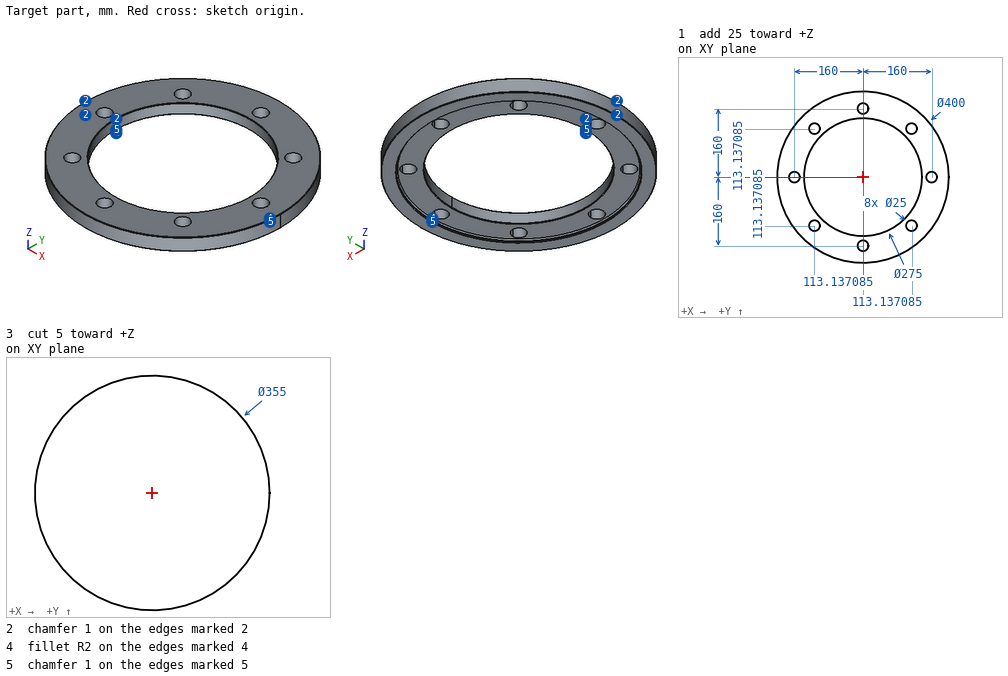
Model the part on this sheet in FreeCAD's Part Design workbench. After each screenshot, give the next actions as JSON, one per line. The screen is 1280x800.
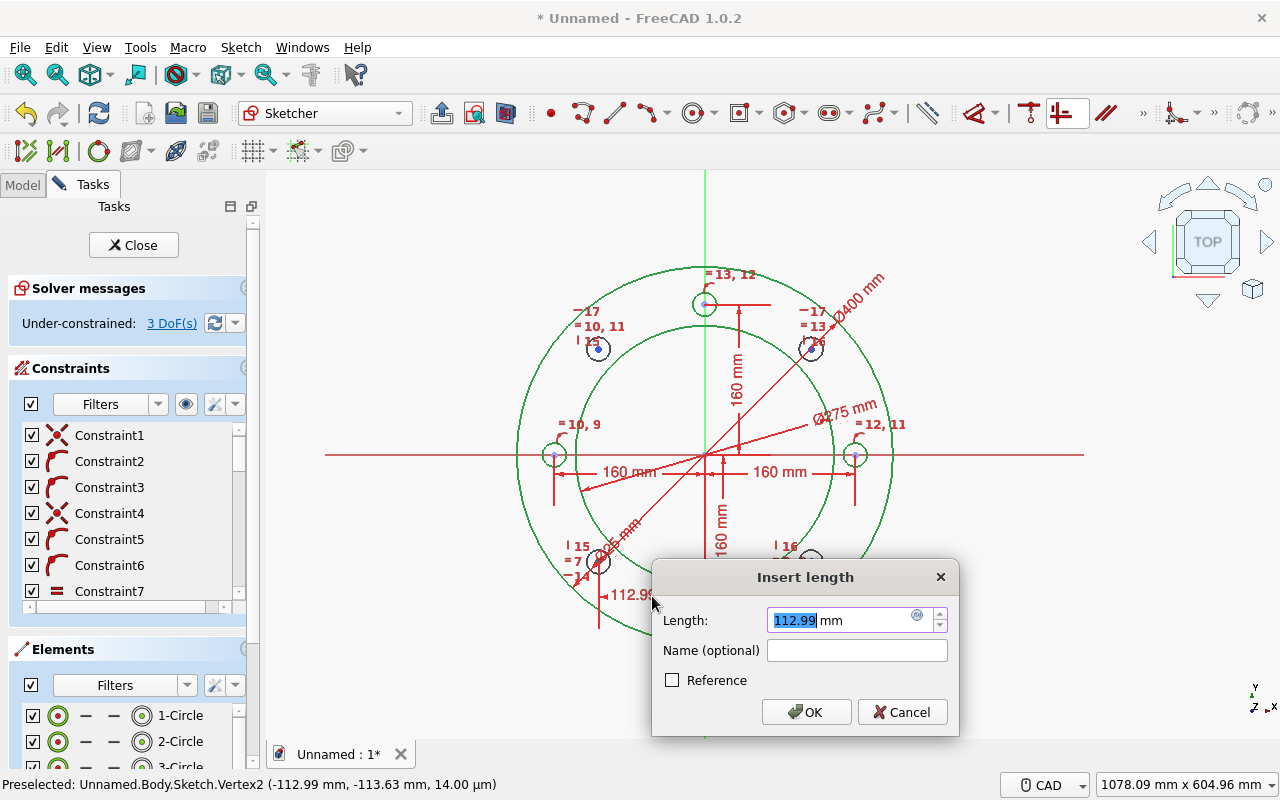
{"action": "type", "text": "113.137085"}
{"action": "key", "text": "Return"}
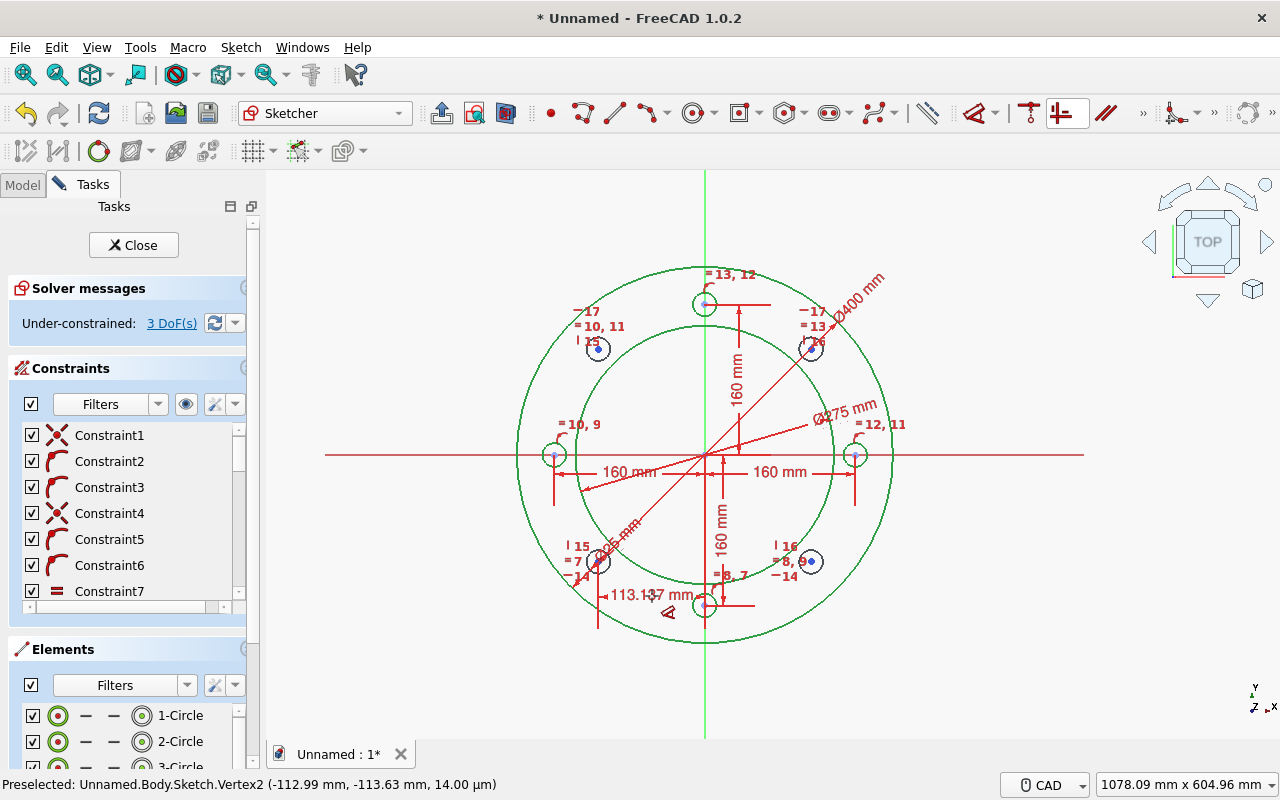
{"action": "left_click", "coordinate": [598, 562]}
{"action": "left_click", "coordinate": [564, 508]}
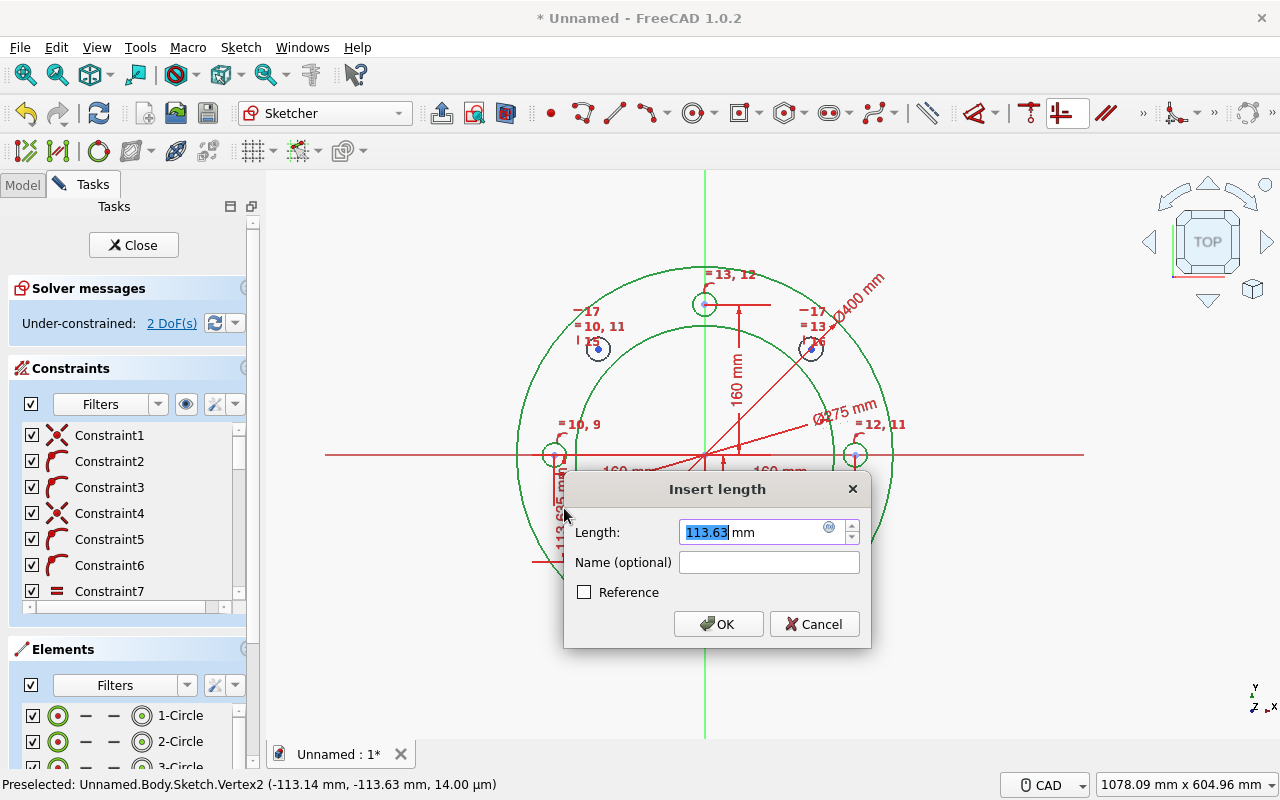
{"action": "type", "text": "113.137085"}
{"action": "key", "text": "Return"}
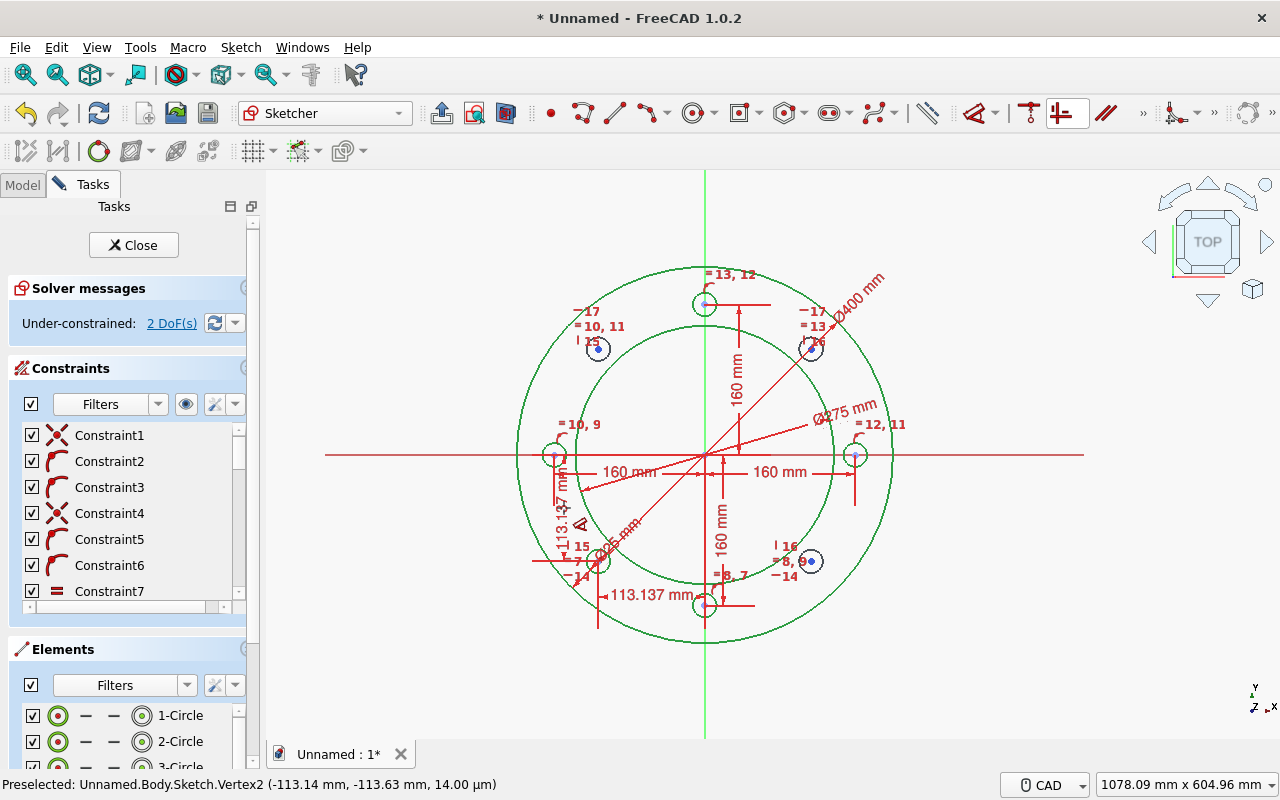
{"action": "left_click", "coordinate": [811, 561]}
{"action": "left_click", "coordinate": [758, 595]}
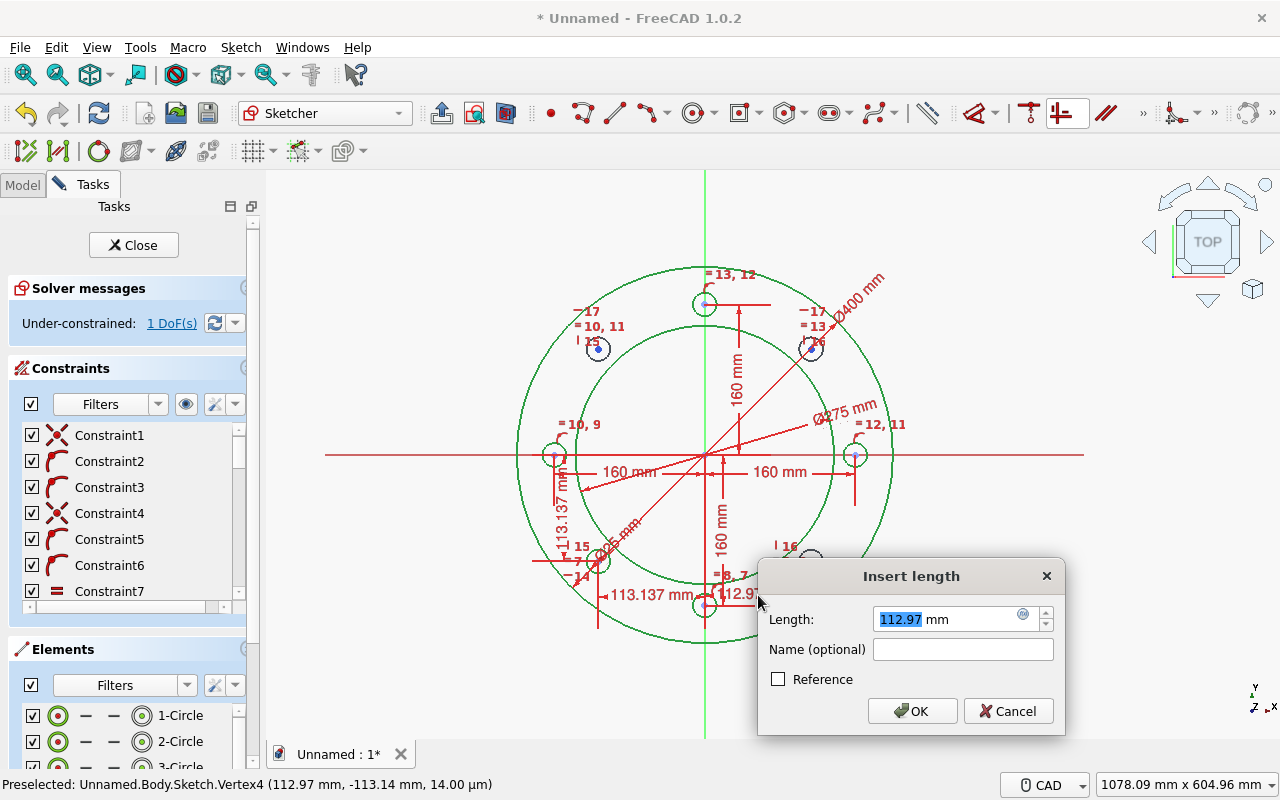
{"action": "type", "text": "113.137085"}
{"action": "key", "text": "Return"}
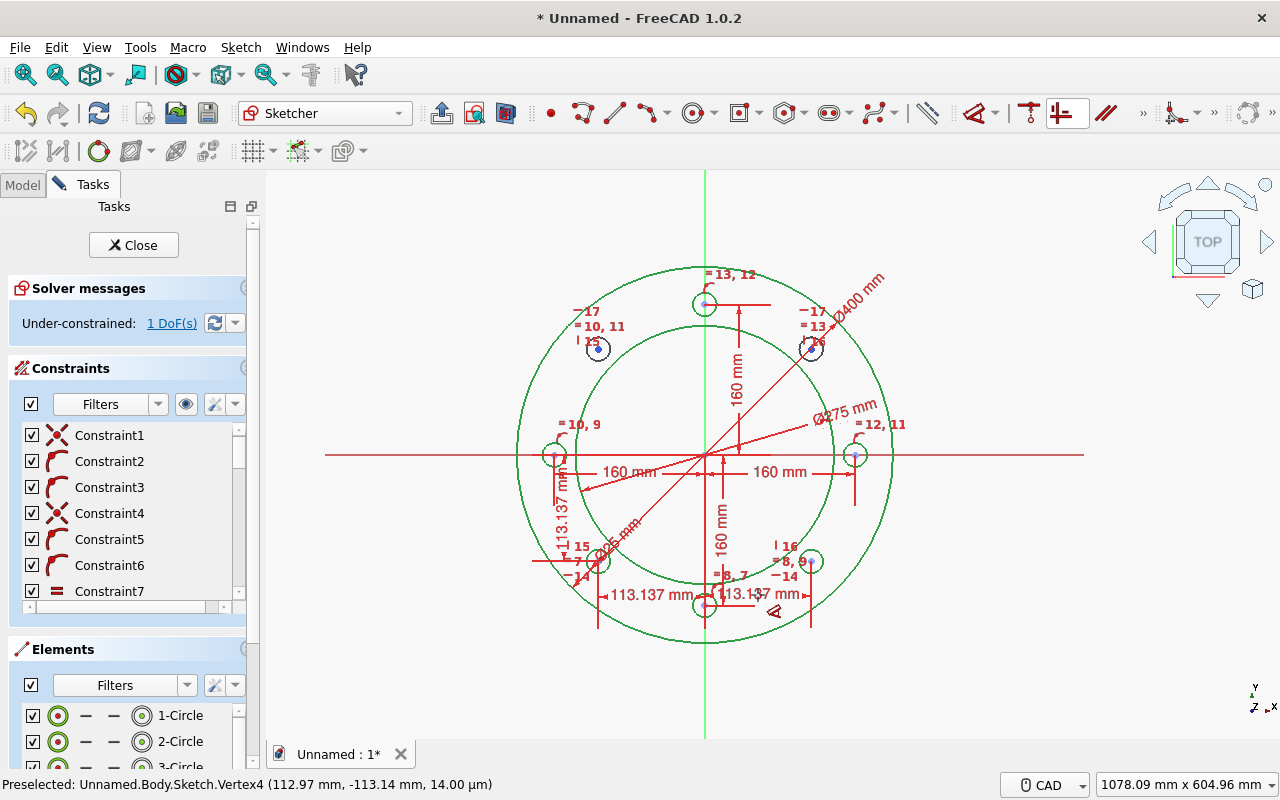
{"action": "left_click", "coordinate": [598, 349]}
{"action": "left_click", "coordinate": [564, 402]}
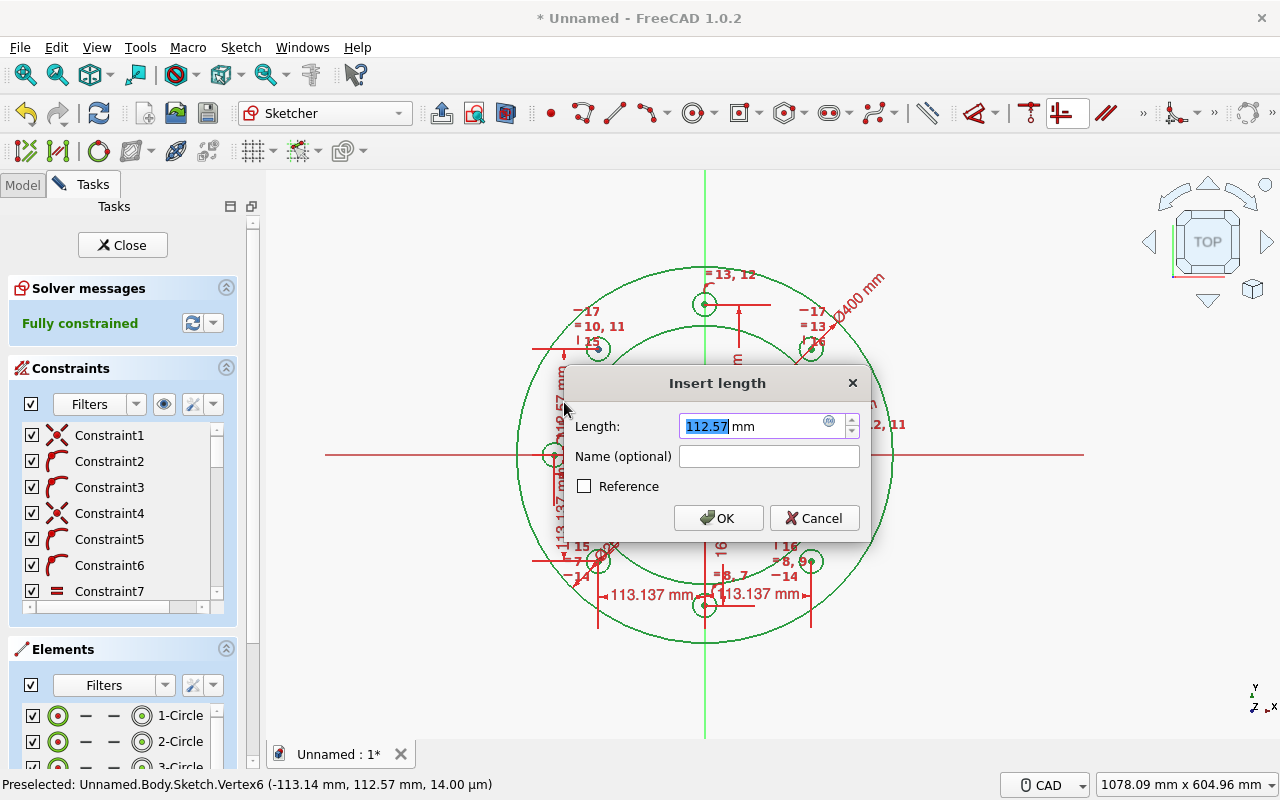
{"action": "type", "text": "113.137085"}
{"action": "key", "text": "Return"}
{"action": "key", "text": "Escape"}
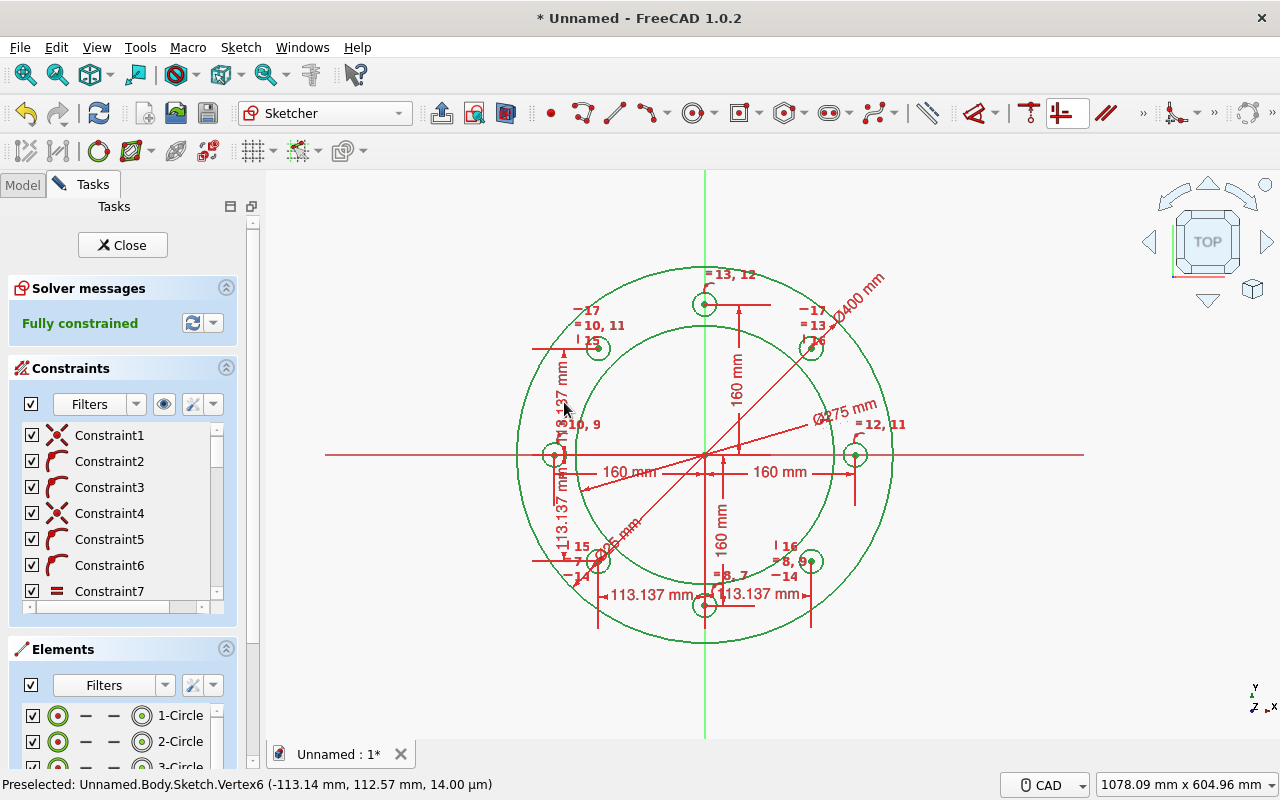
{"action": "left_click", "coordinate": [123, 245]}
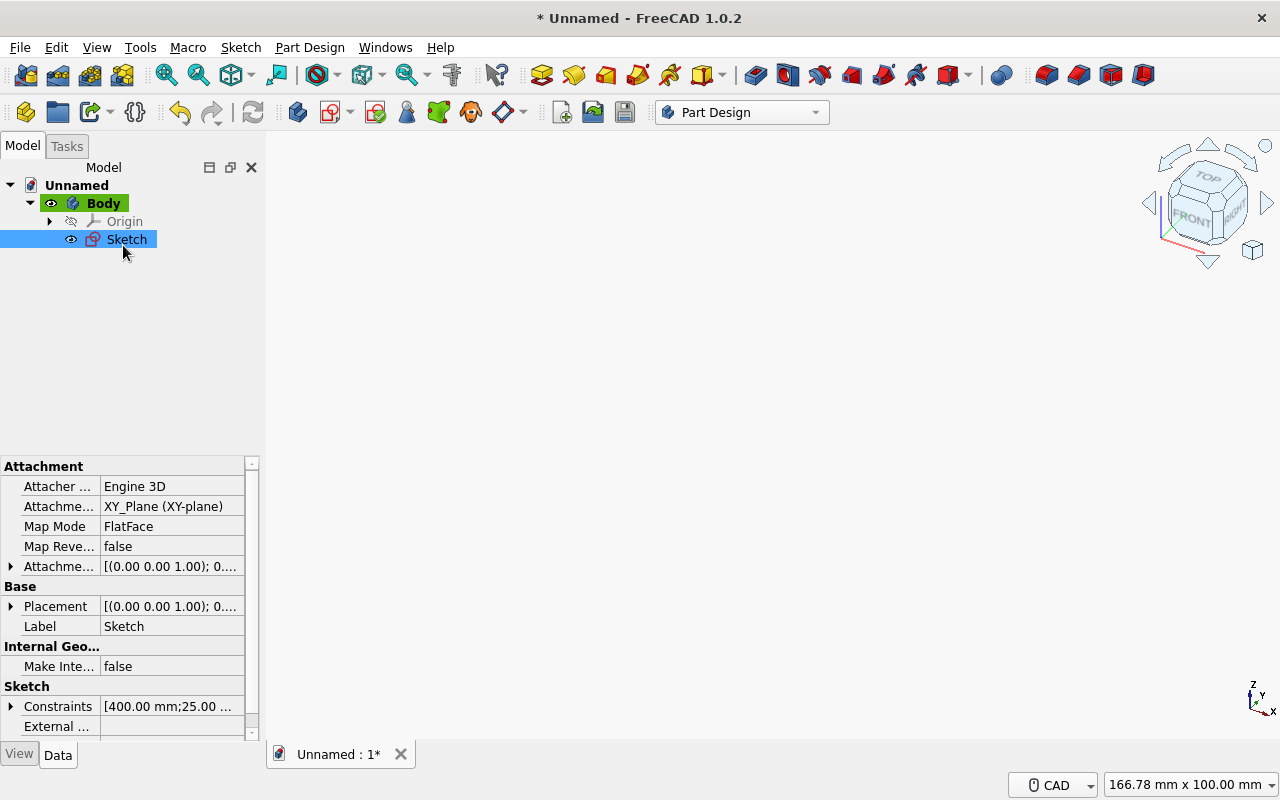
{"action": "left_click", "coordinate": [542, 76]}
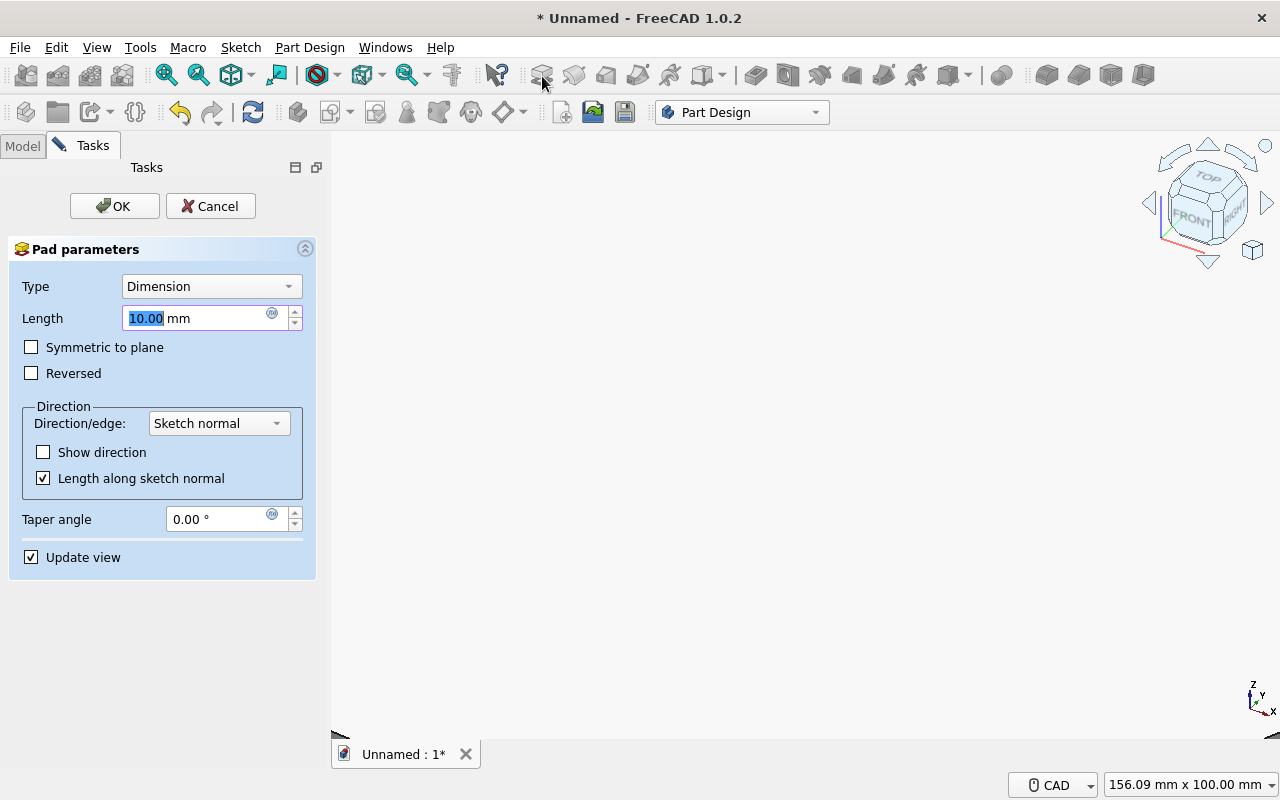
{"action": "type", "text": "25"}
{"action": "key", "text": "Tab"}